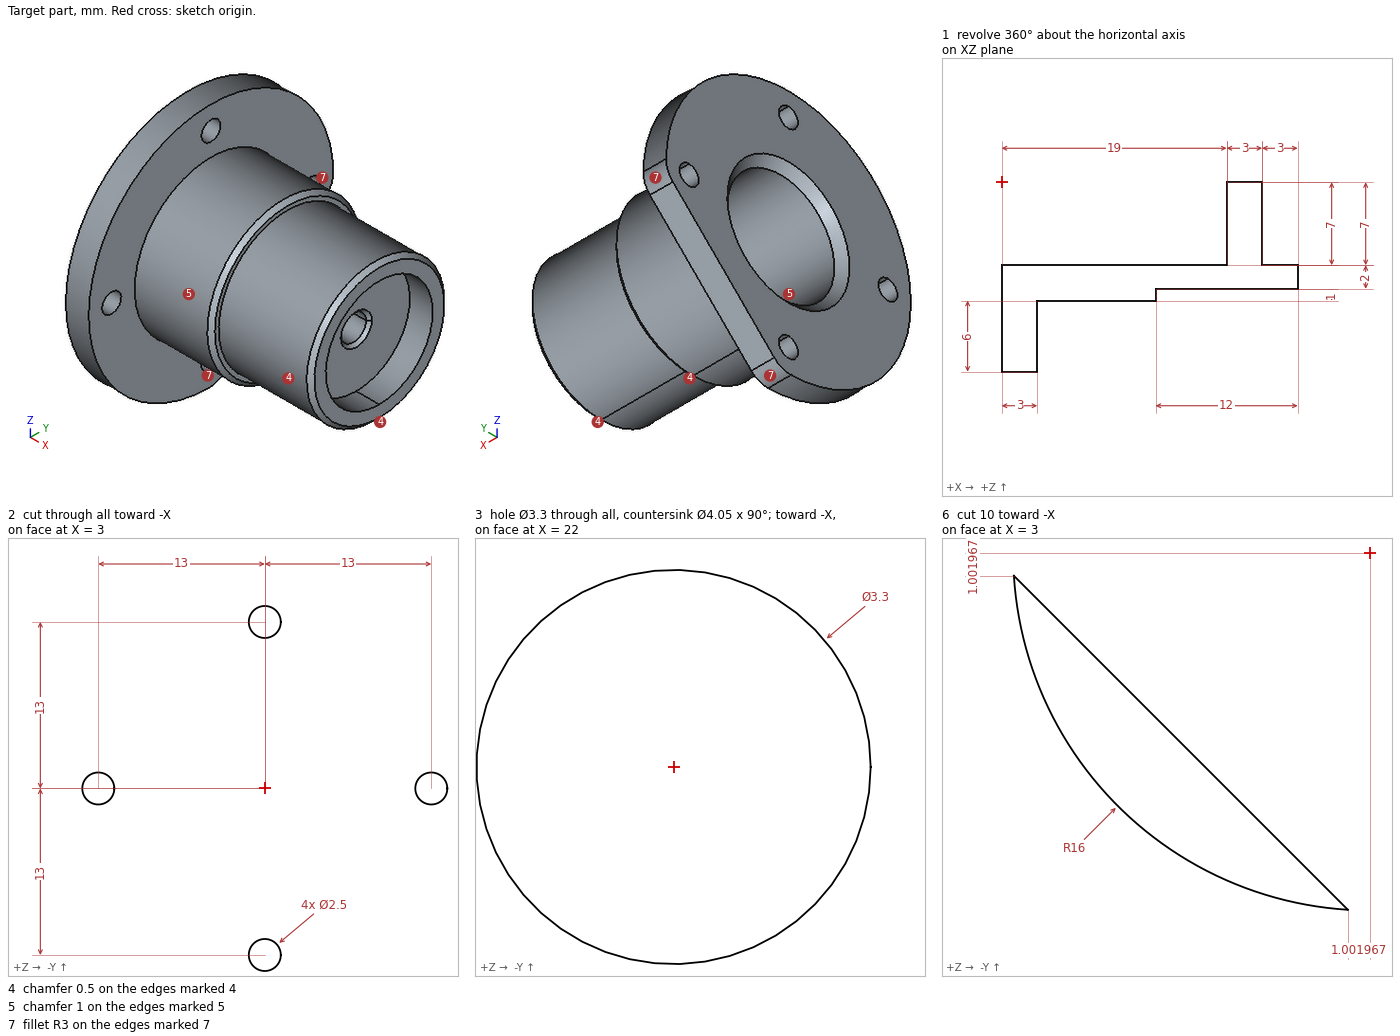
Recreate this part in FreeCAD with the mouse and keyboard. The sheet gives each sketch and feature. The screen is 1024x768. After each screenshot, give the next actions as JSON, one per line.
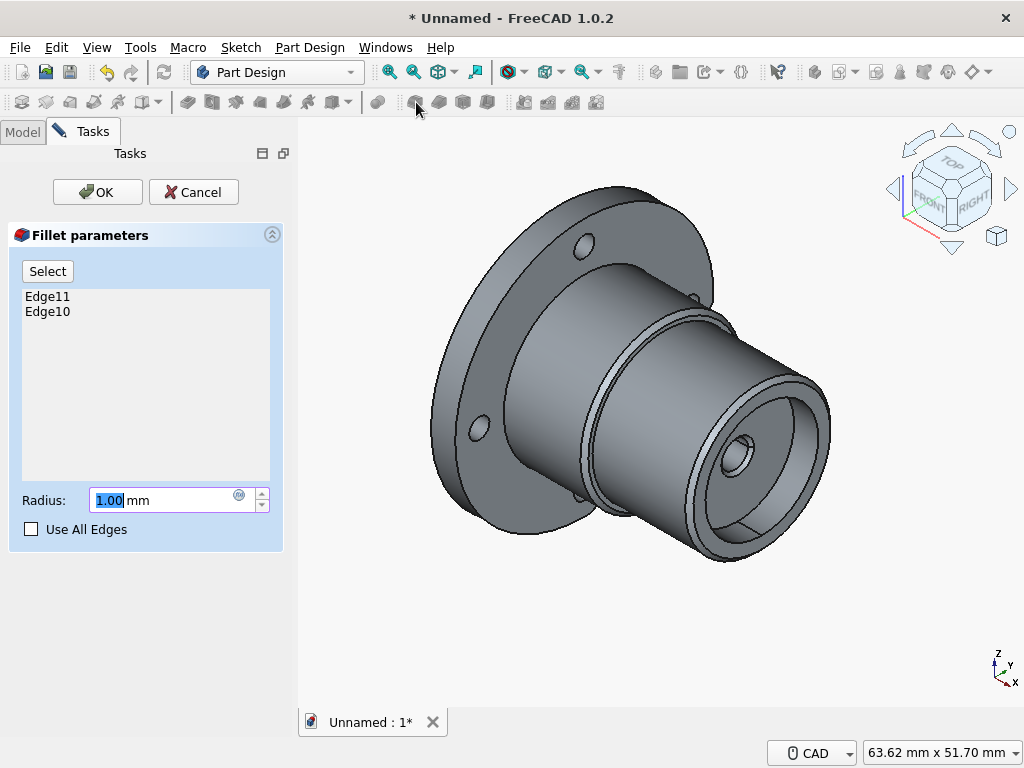
{"action": "type", "text": "3"}
{"action": "key", "text": "Tab"}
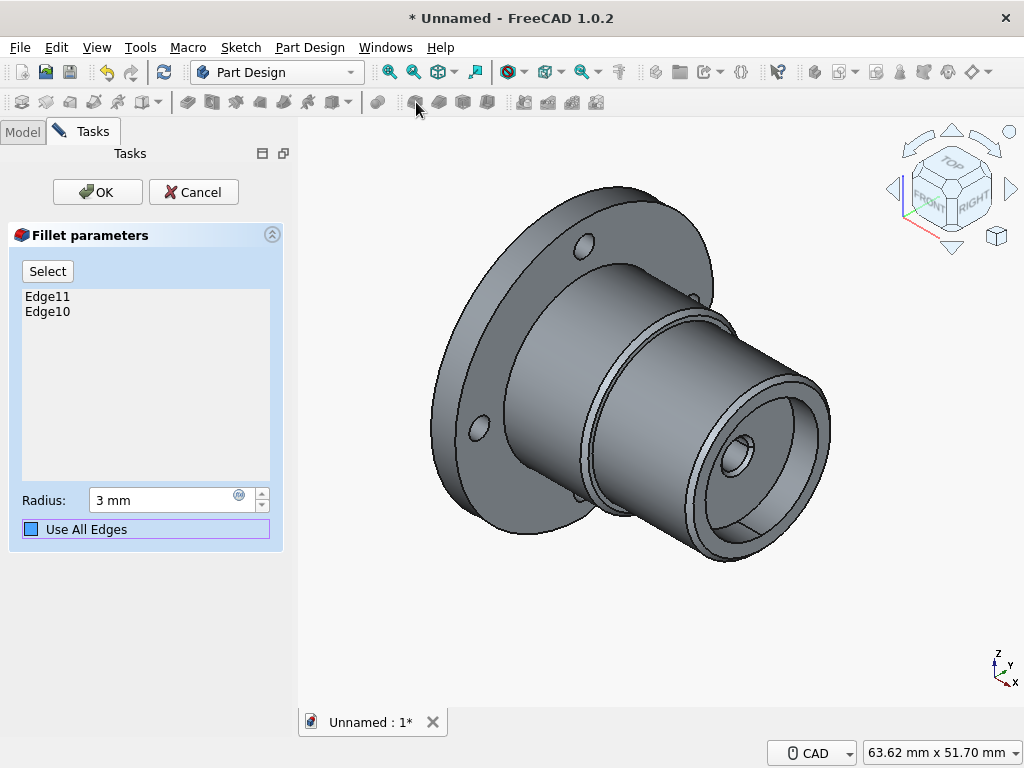
{"action": "left_click", "coordinate": [98, 192]}